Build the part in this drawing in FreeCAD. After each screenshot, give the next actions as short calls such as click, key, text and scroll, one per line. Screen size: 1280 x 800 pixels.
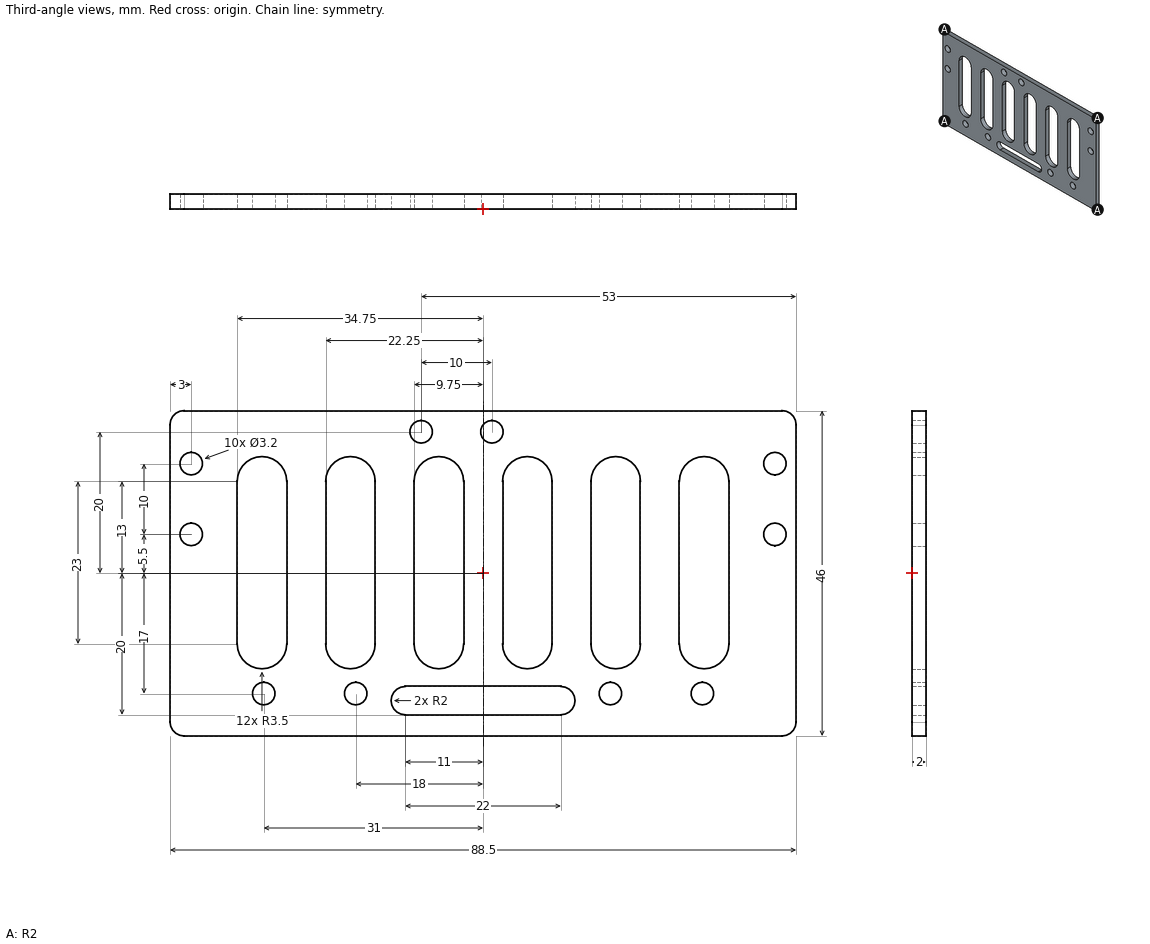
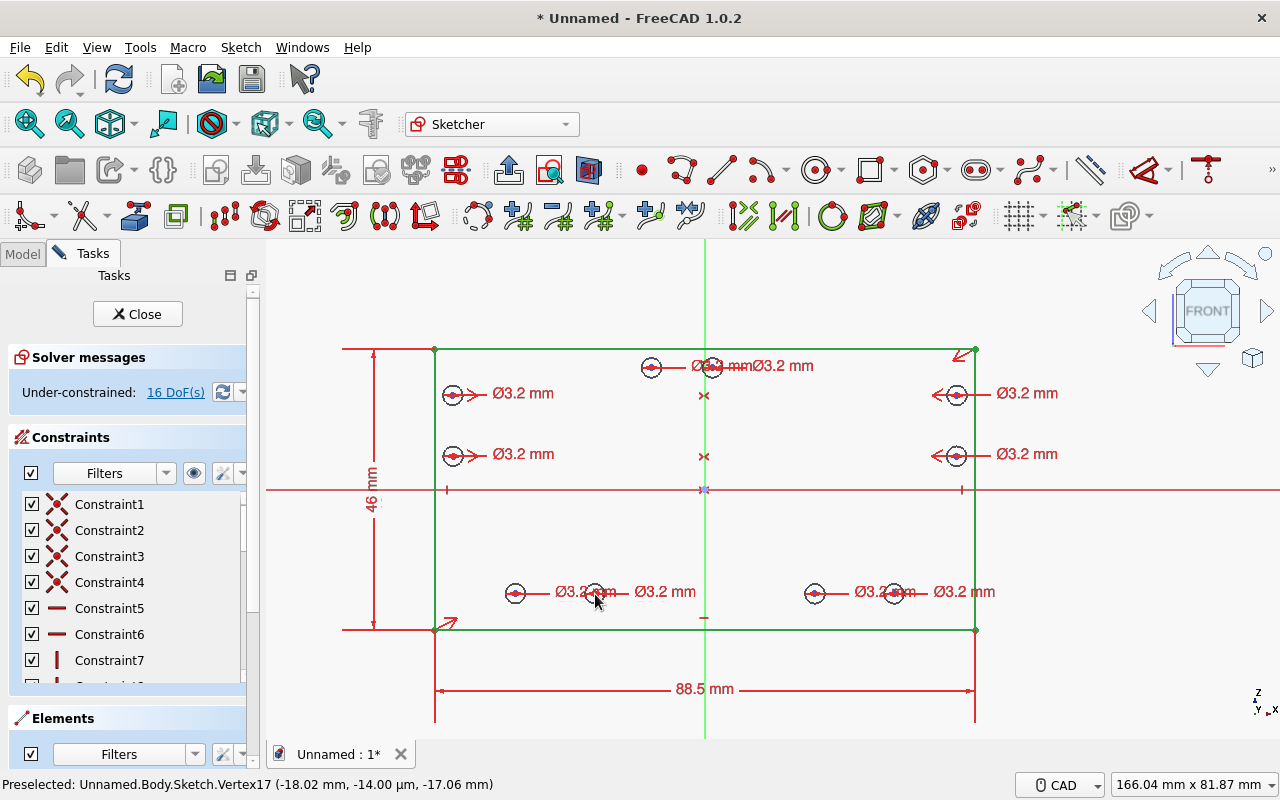
click(815, 594)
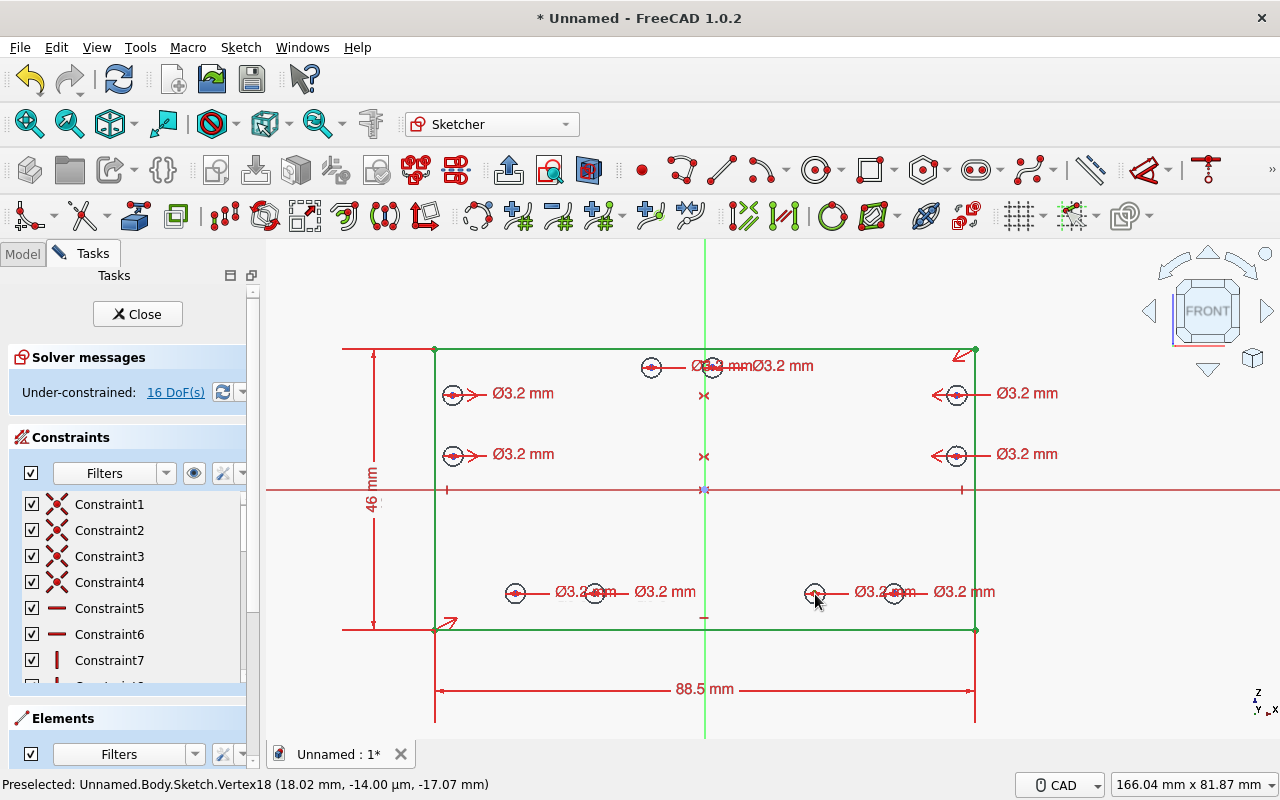
click(705, 679)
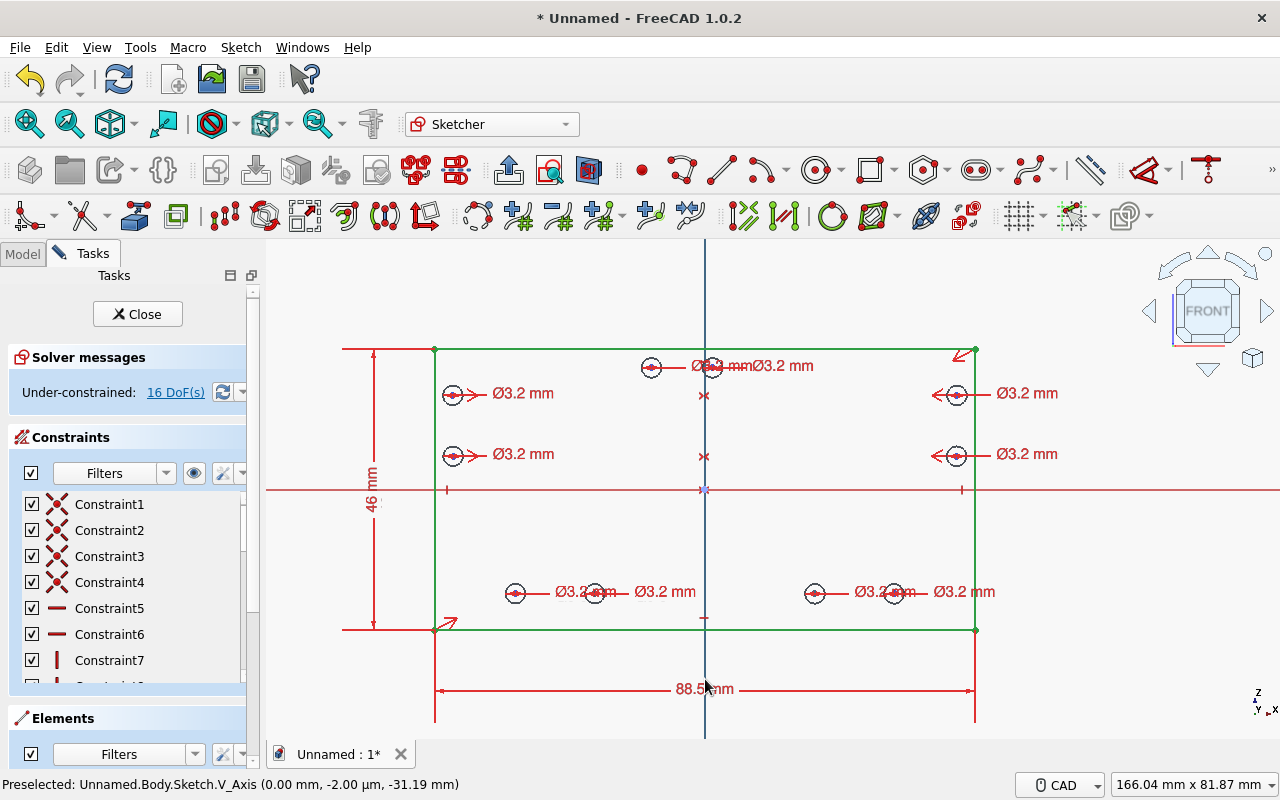
key(s)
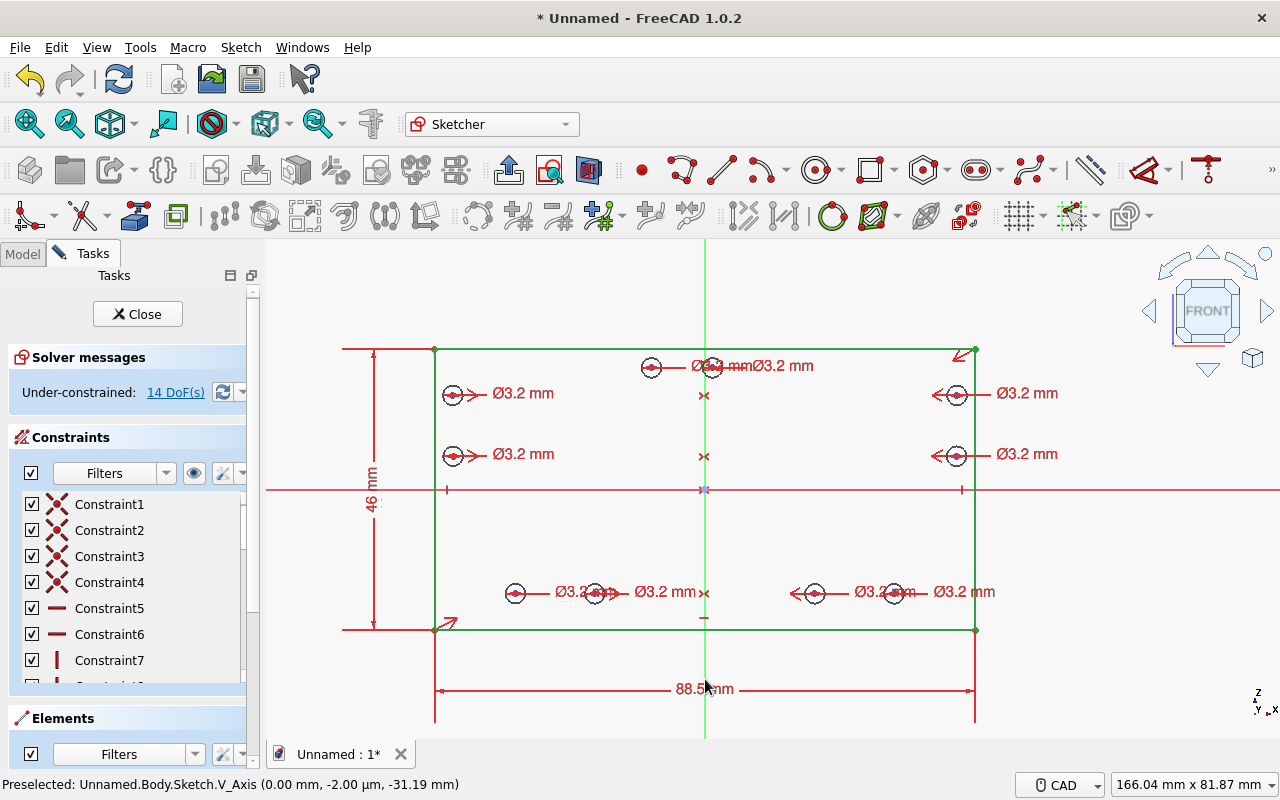
click(515, 594)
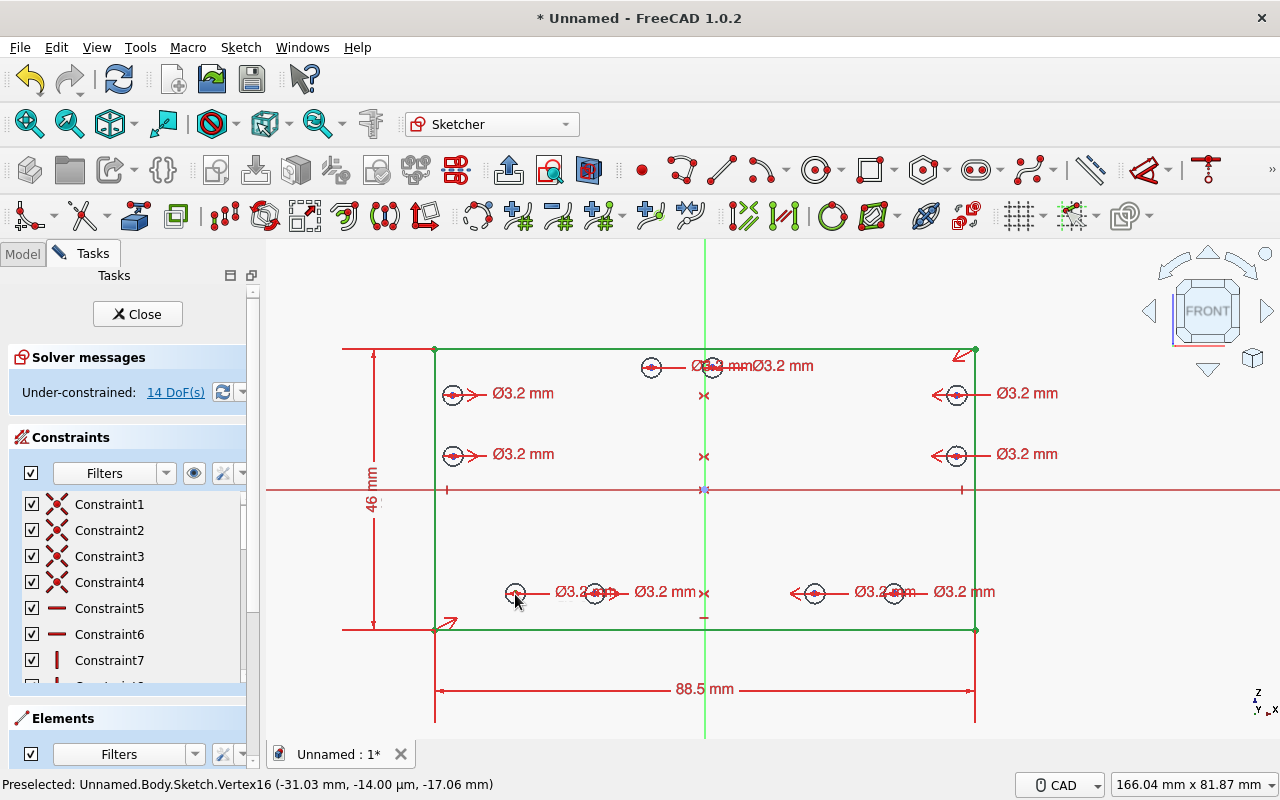
click(894, 594)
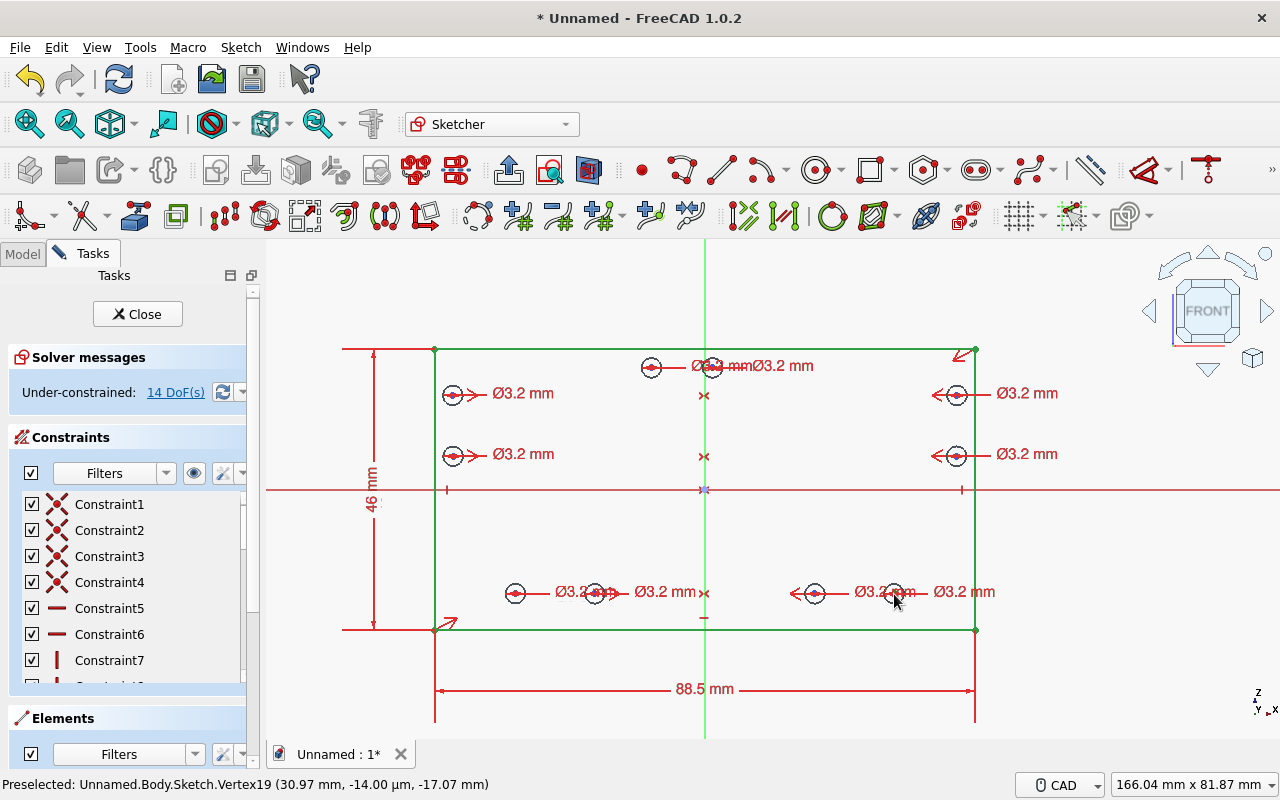
click(705, 679)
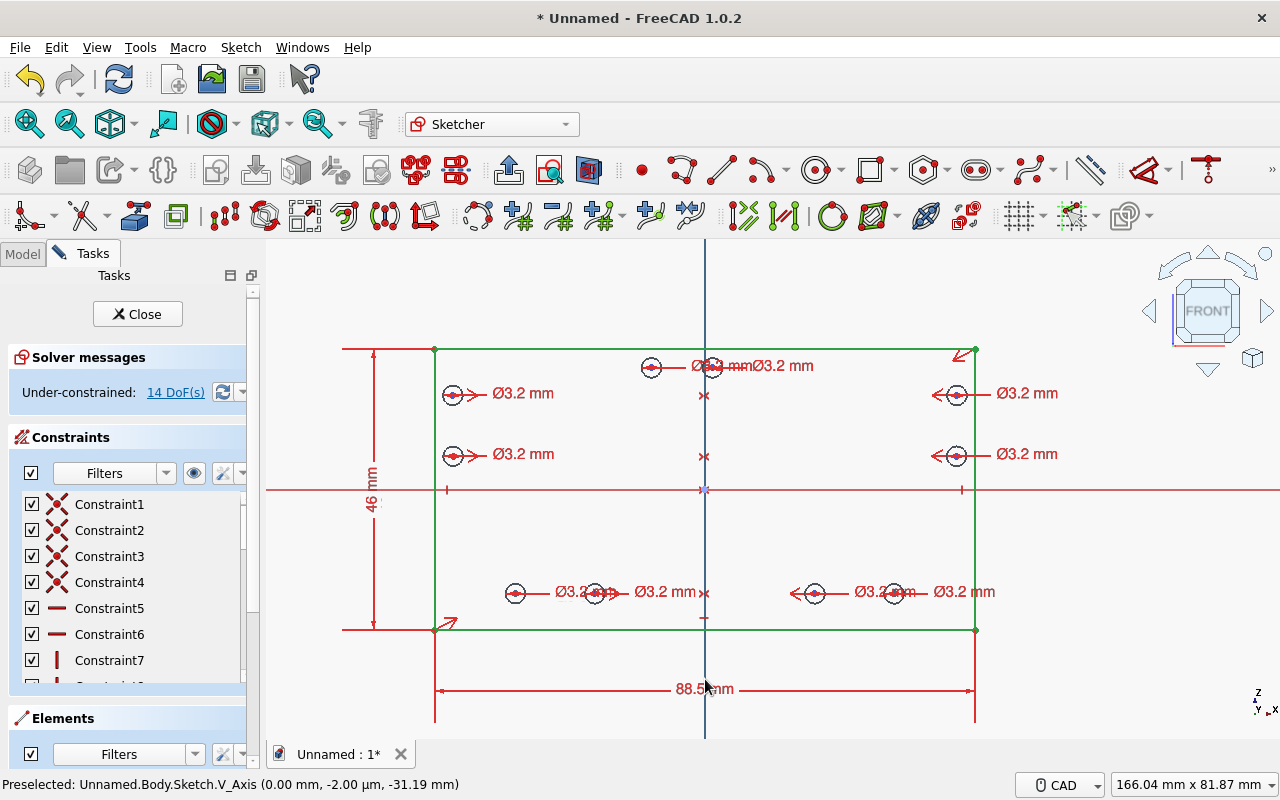
key(s)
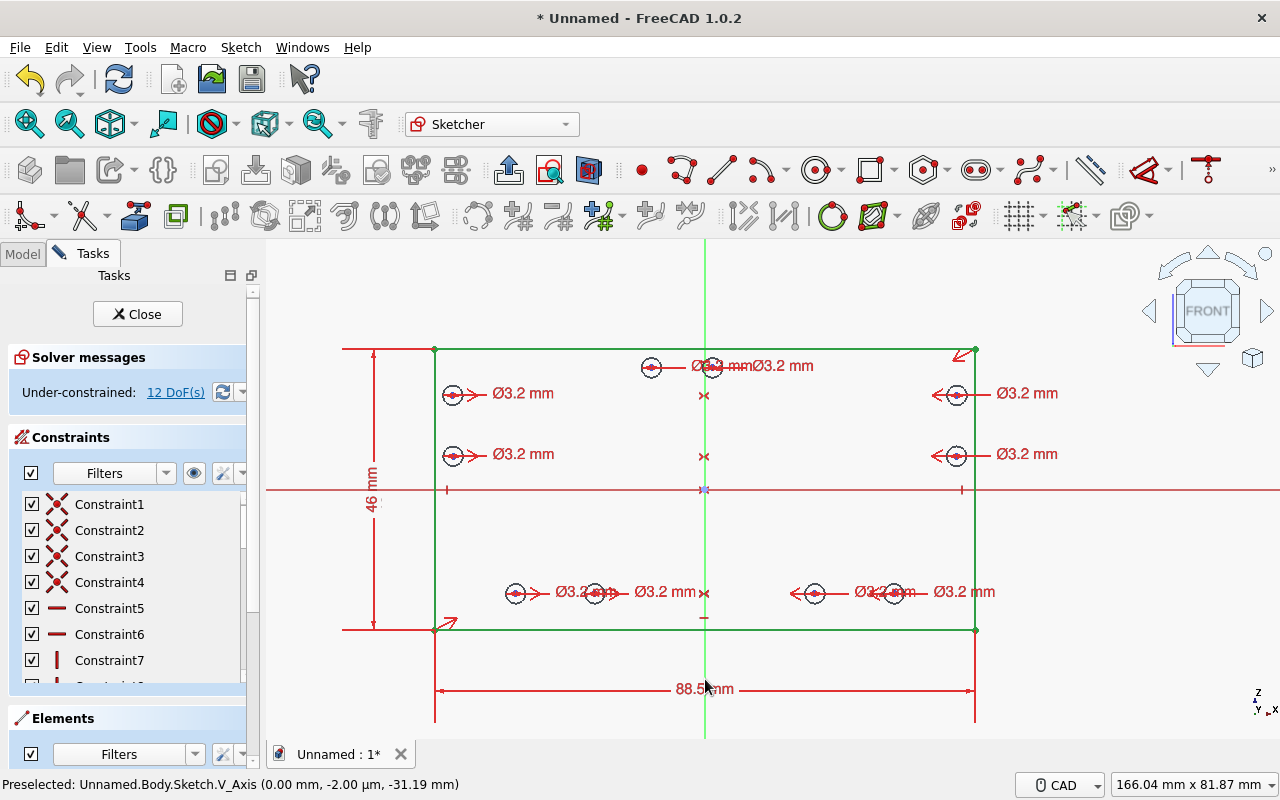
click(1144, 170)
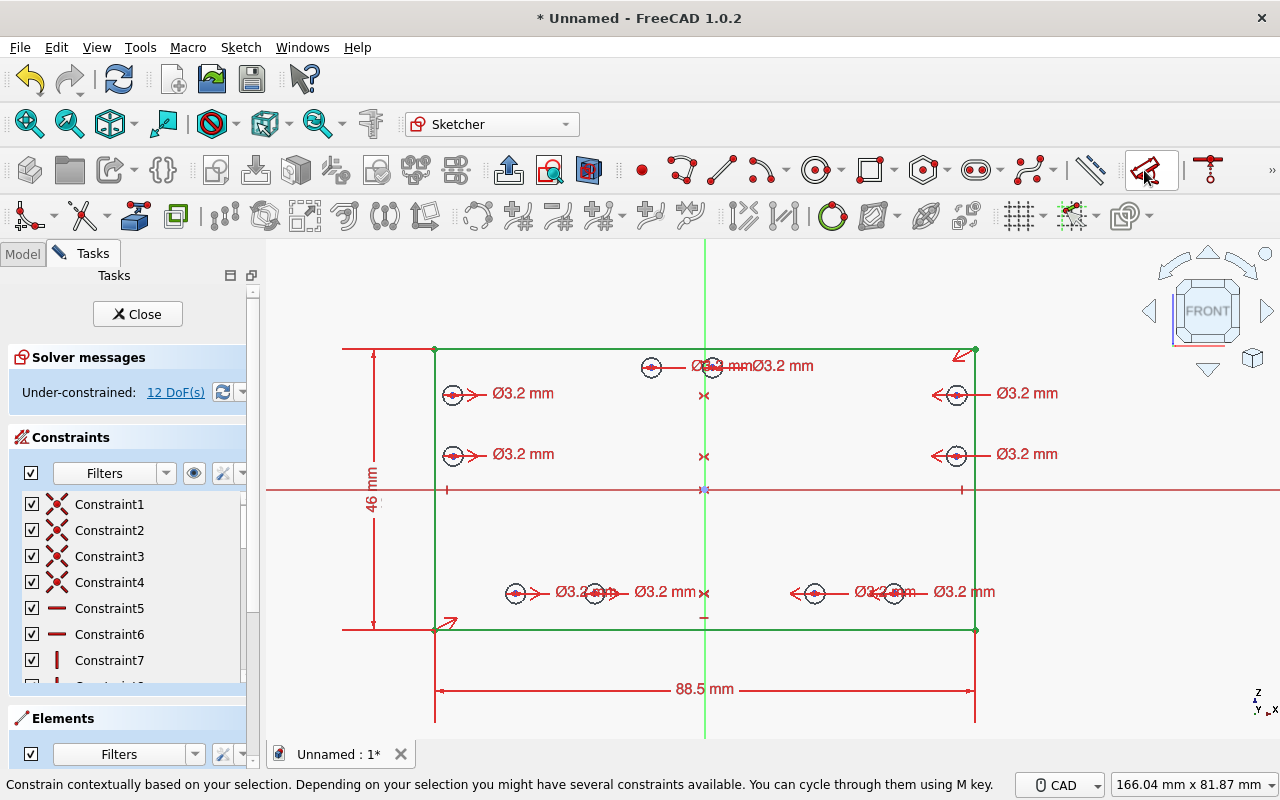
click(651, 368)
click(617, 429)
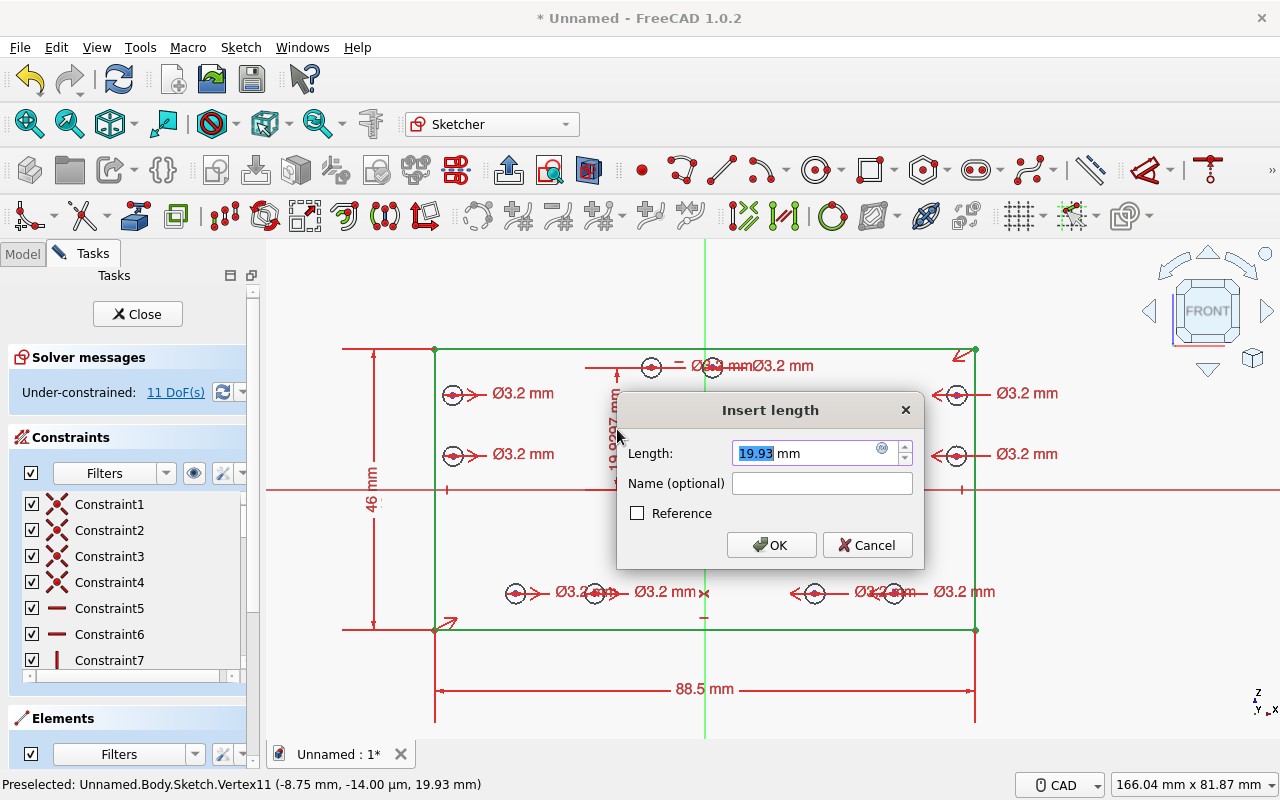
text(20)
key(Return)